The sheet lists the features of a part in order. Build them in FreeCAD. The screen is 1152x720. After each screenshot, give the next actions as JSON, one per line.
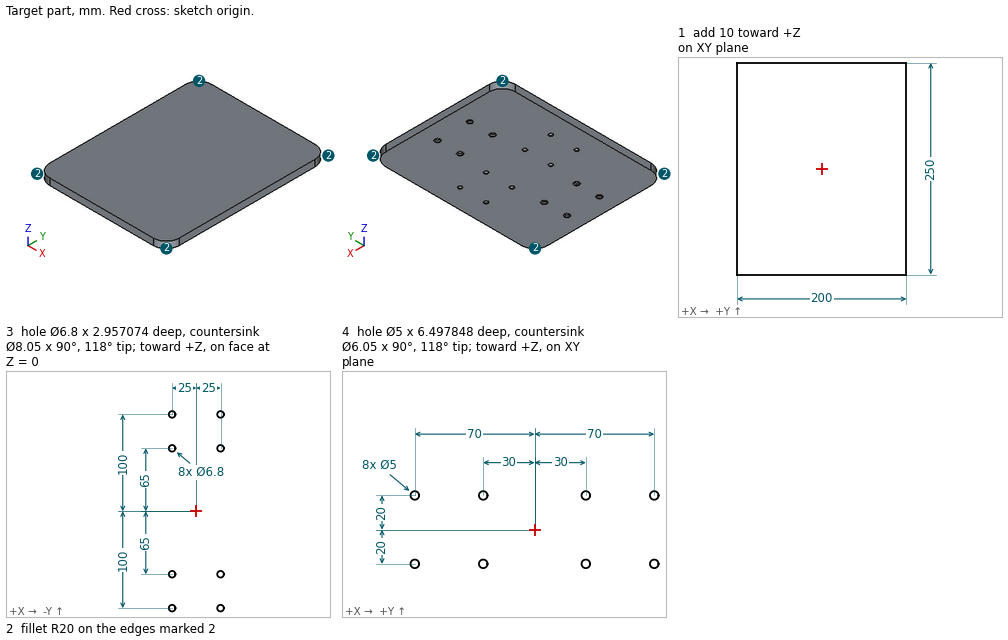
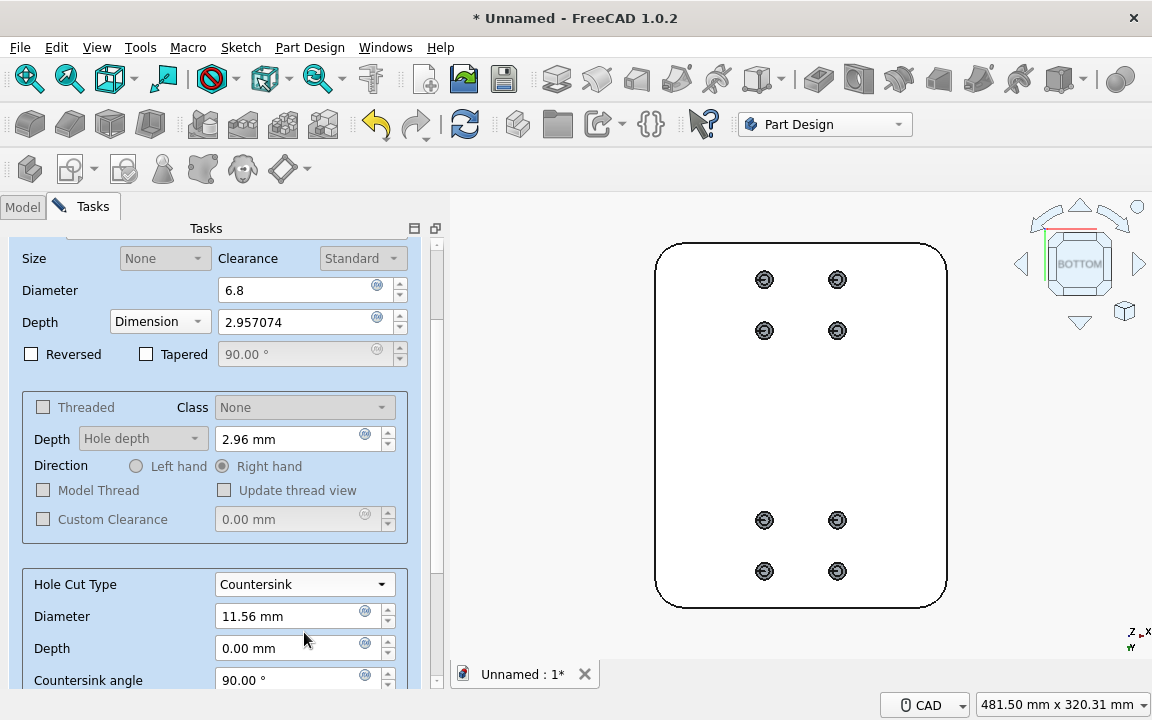
{"action": "triple_click", "coordinate": [298, 616]}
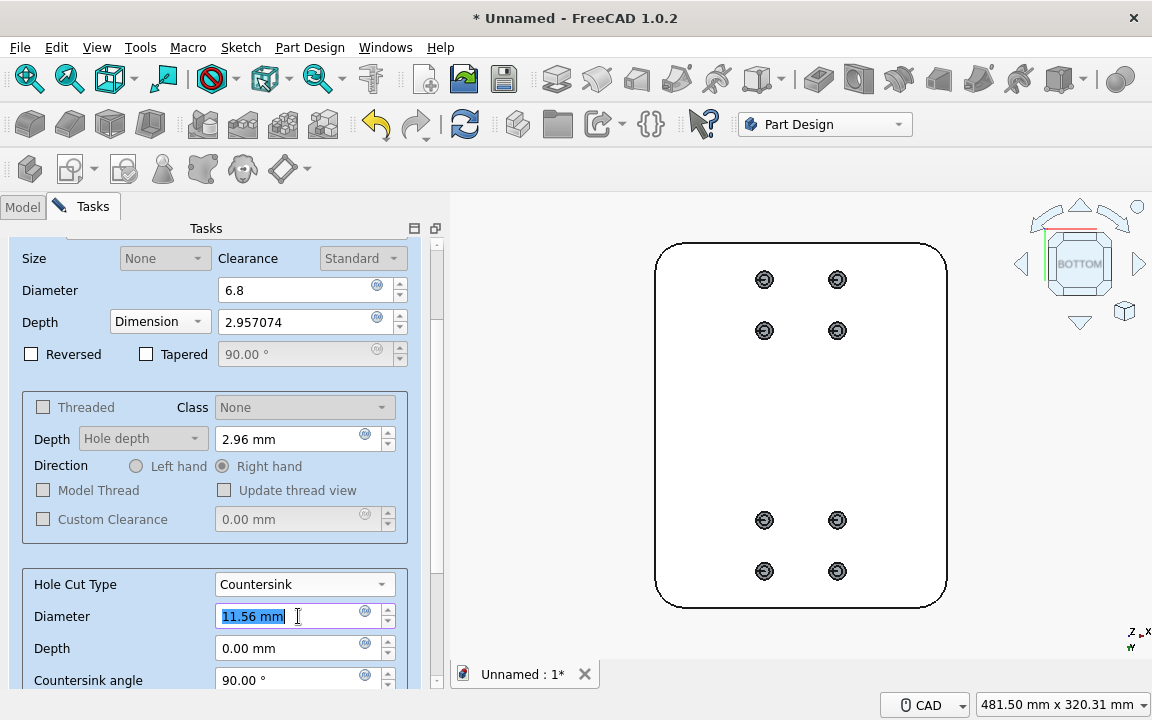
{"action": "type", "text": "8.05"}
{"action": "key", "text": "Tab"}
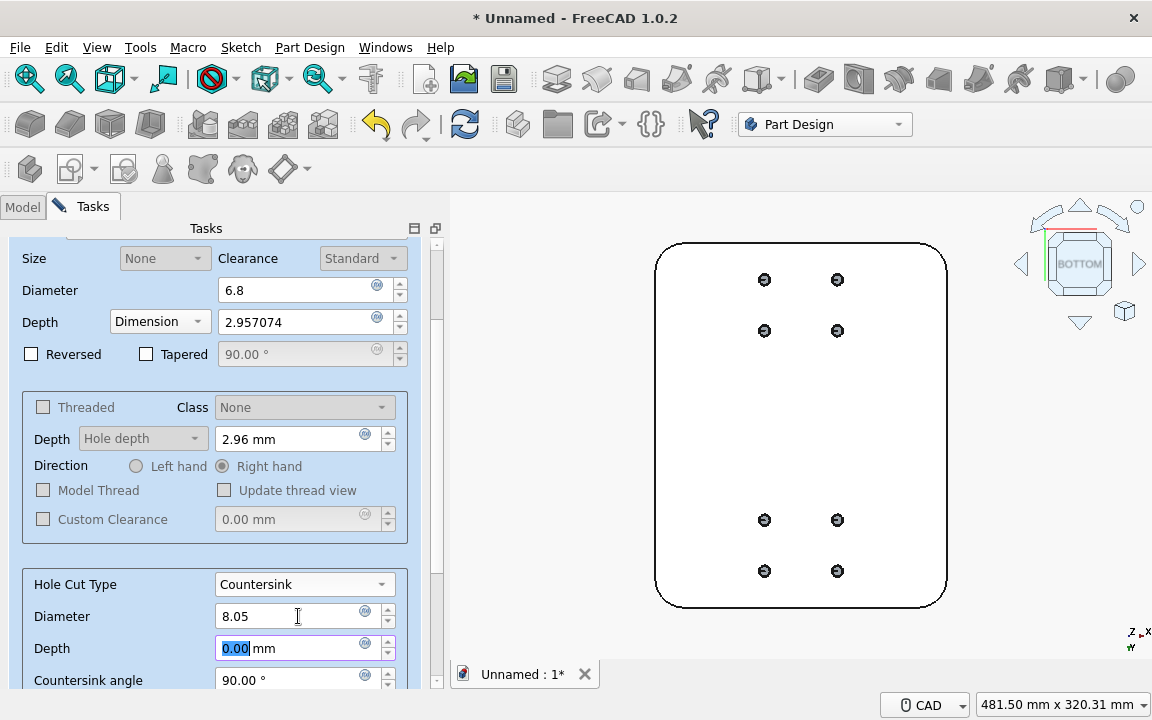
{"action": "scroll", "coordinate": [437, 463], "scroll_direction": "up", "scroll_amount": 3}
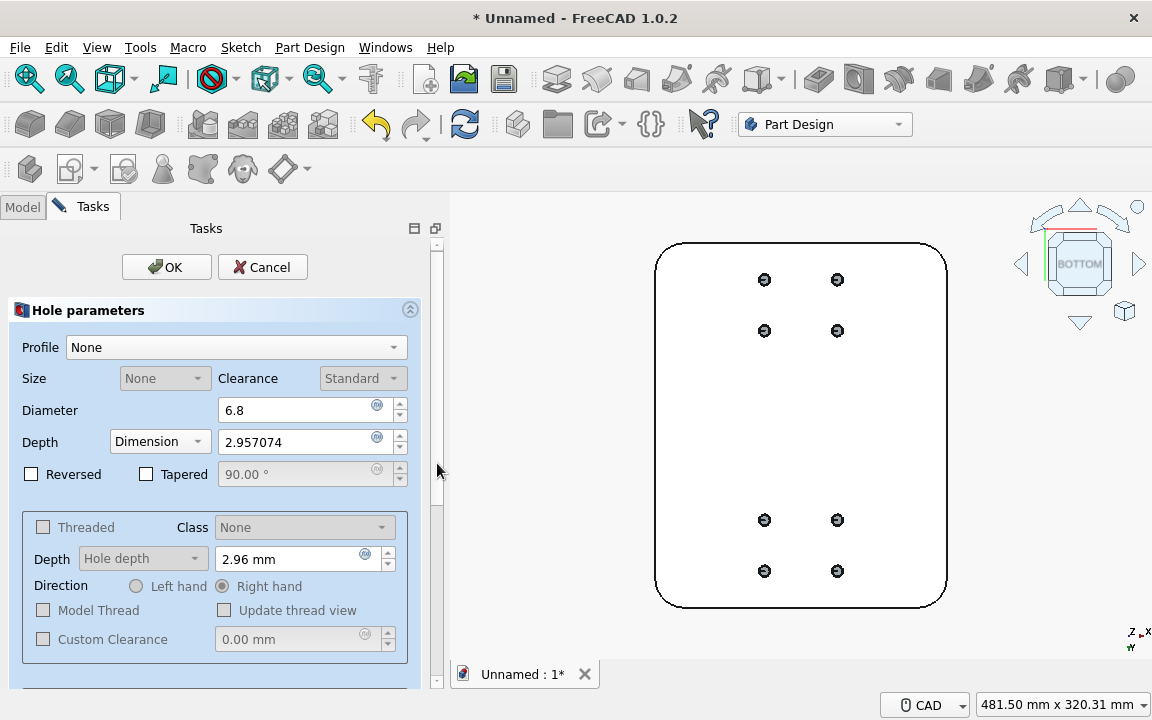
{"action": "left_click", "coordinate": [167, 267]}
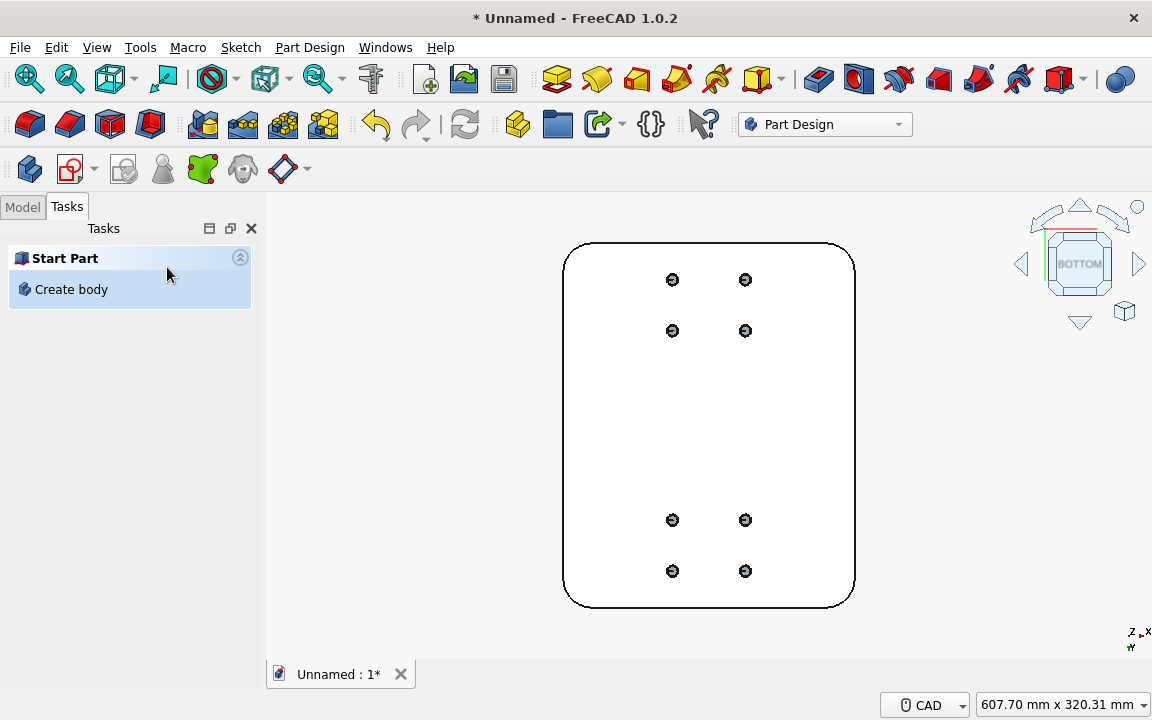
{"action": "left_click", "coordinate": [70, 170]}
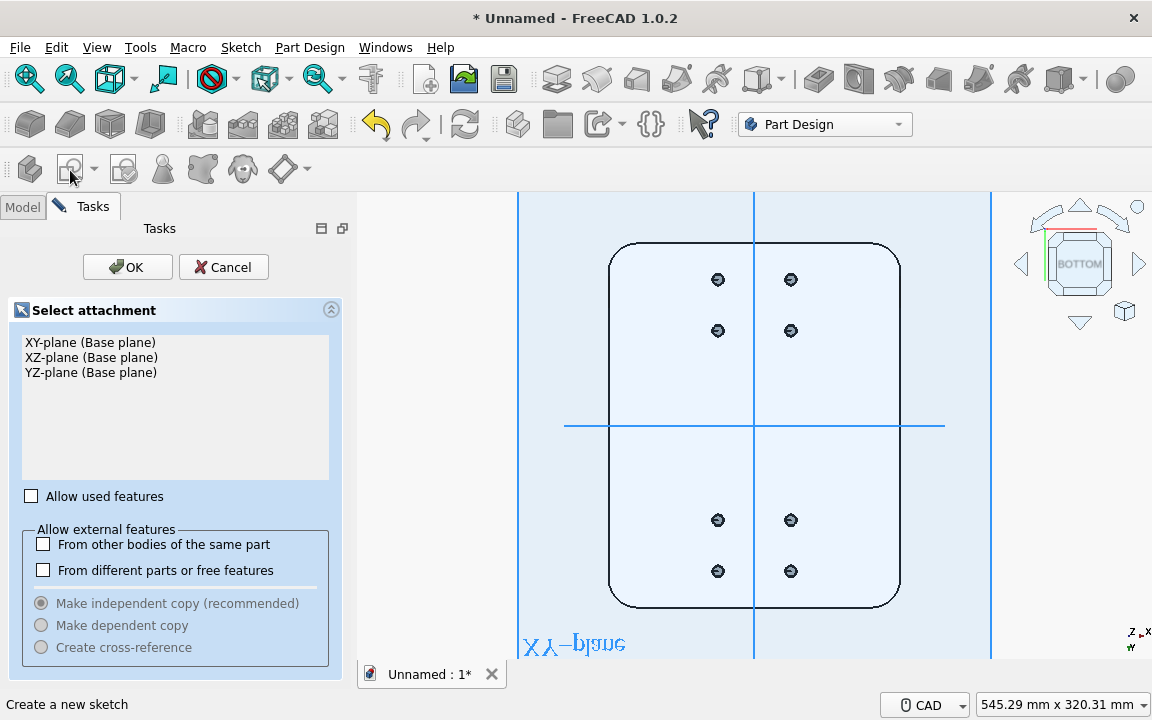
{"action": "left_click", "coordinate": [82, 342]}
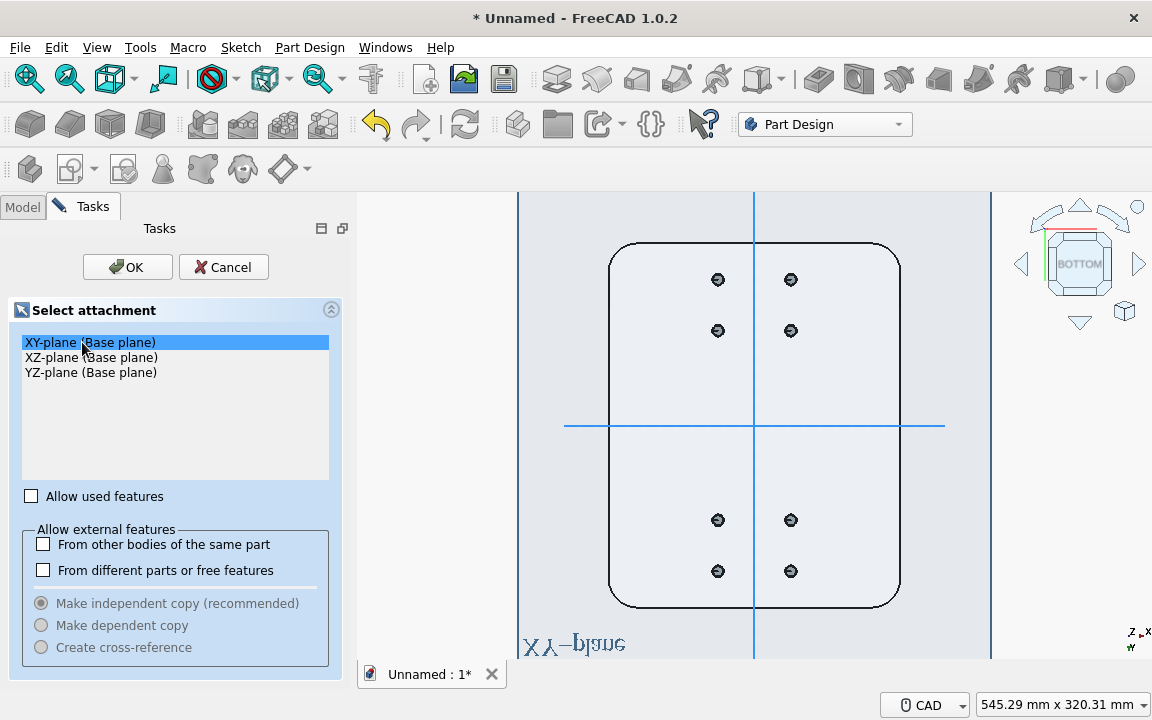
{"action": "left_click", "coordinate": [128, 267]}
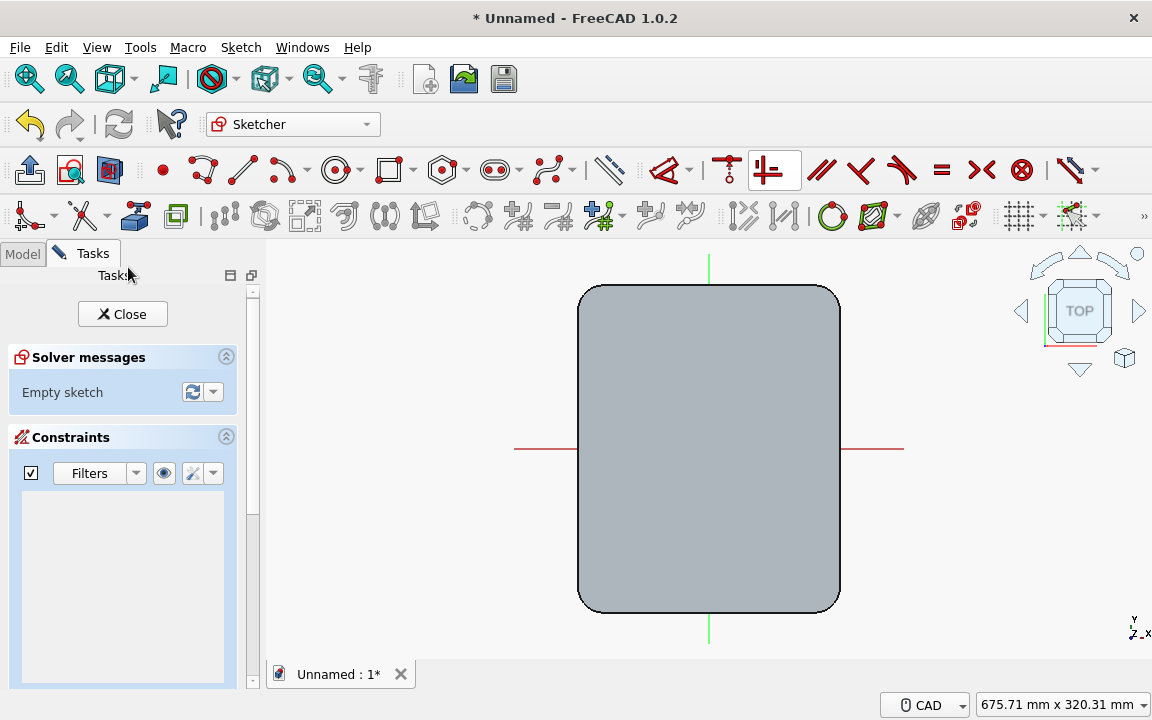
{"action": "key", "text": "q s"}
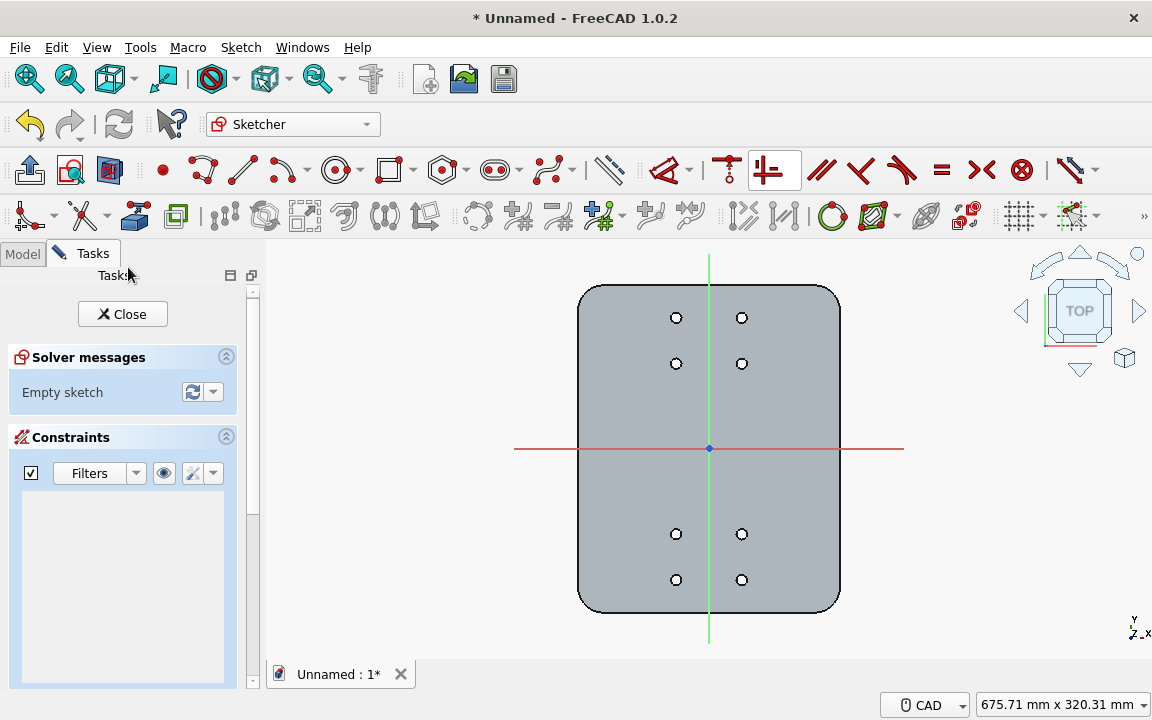
{"action": "scroll", "coordinate": [749, 449], "scroll_direction": "up", "scroll_amount": 5}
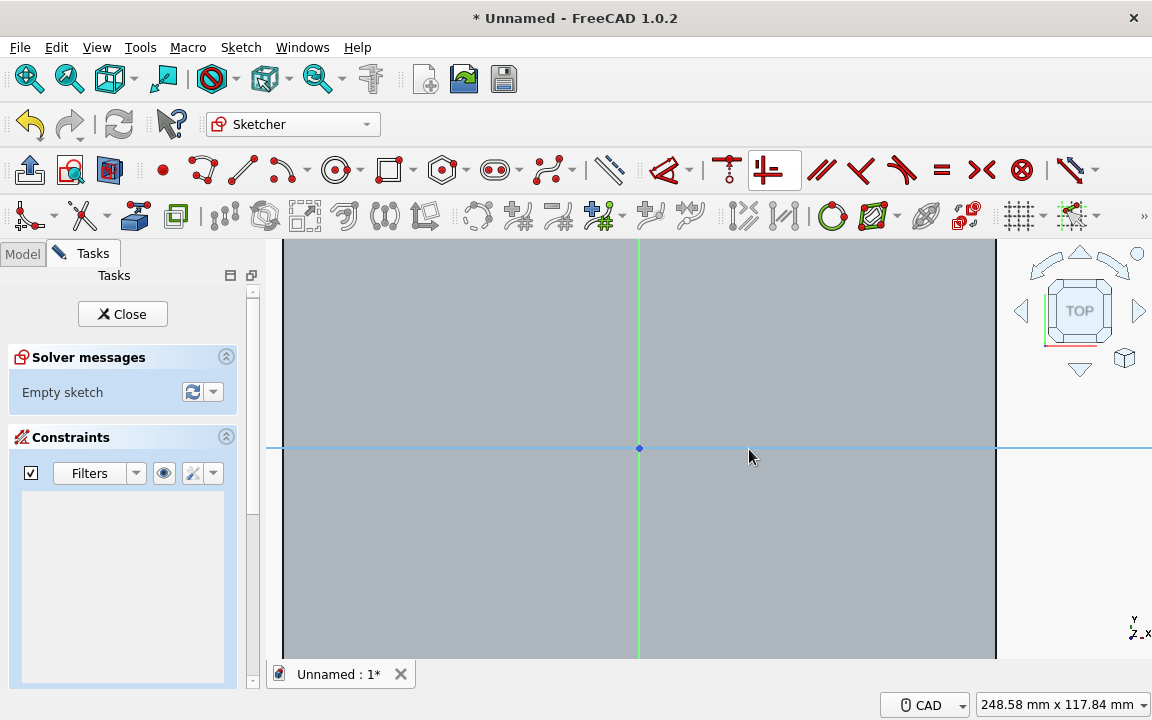
{"action": "key", "text": "g c"}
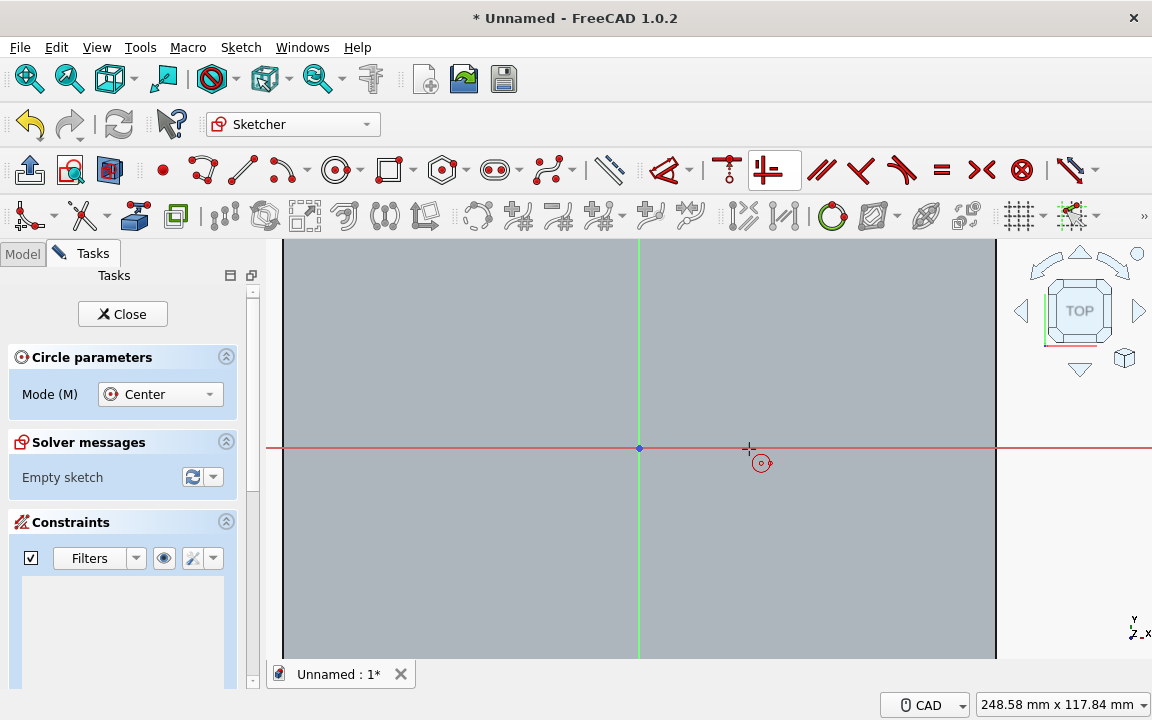
{"action": "scroll", "coordinate": [390, 377], "scroll_direction": "up", "scroll_amount": 5}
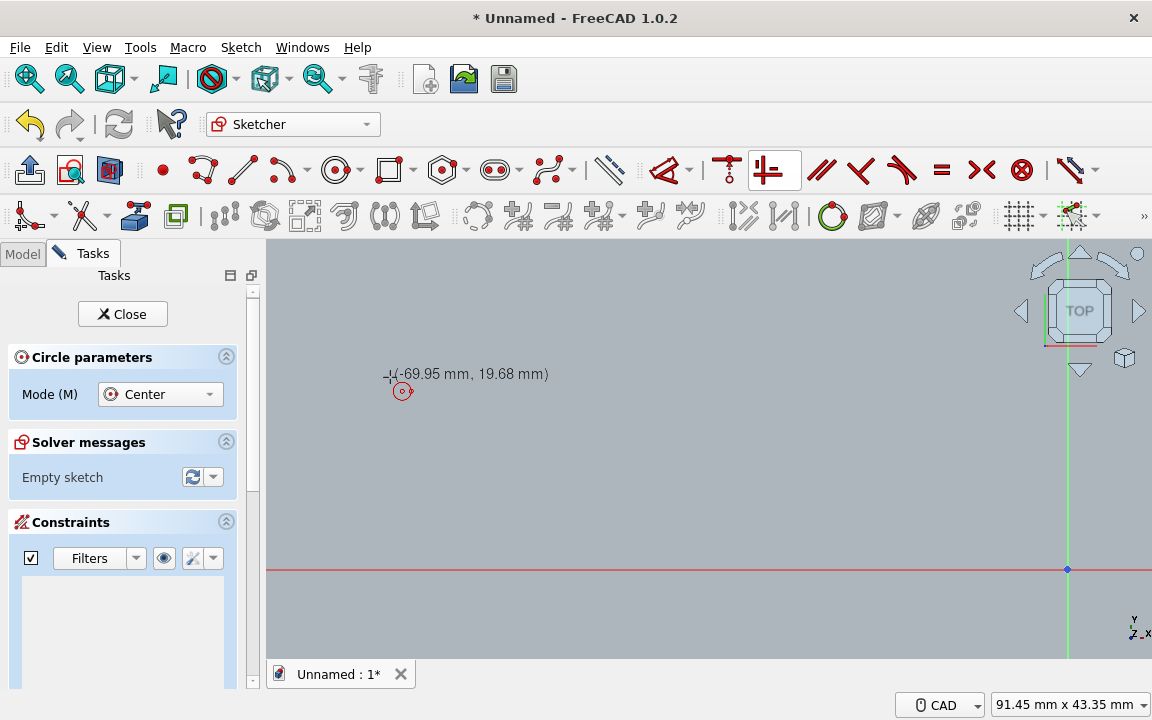
{"action": "left_click", "coordinate": [389, 376]}
{"action": "mouse_move", "coordinate": [406, 359]}